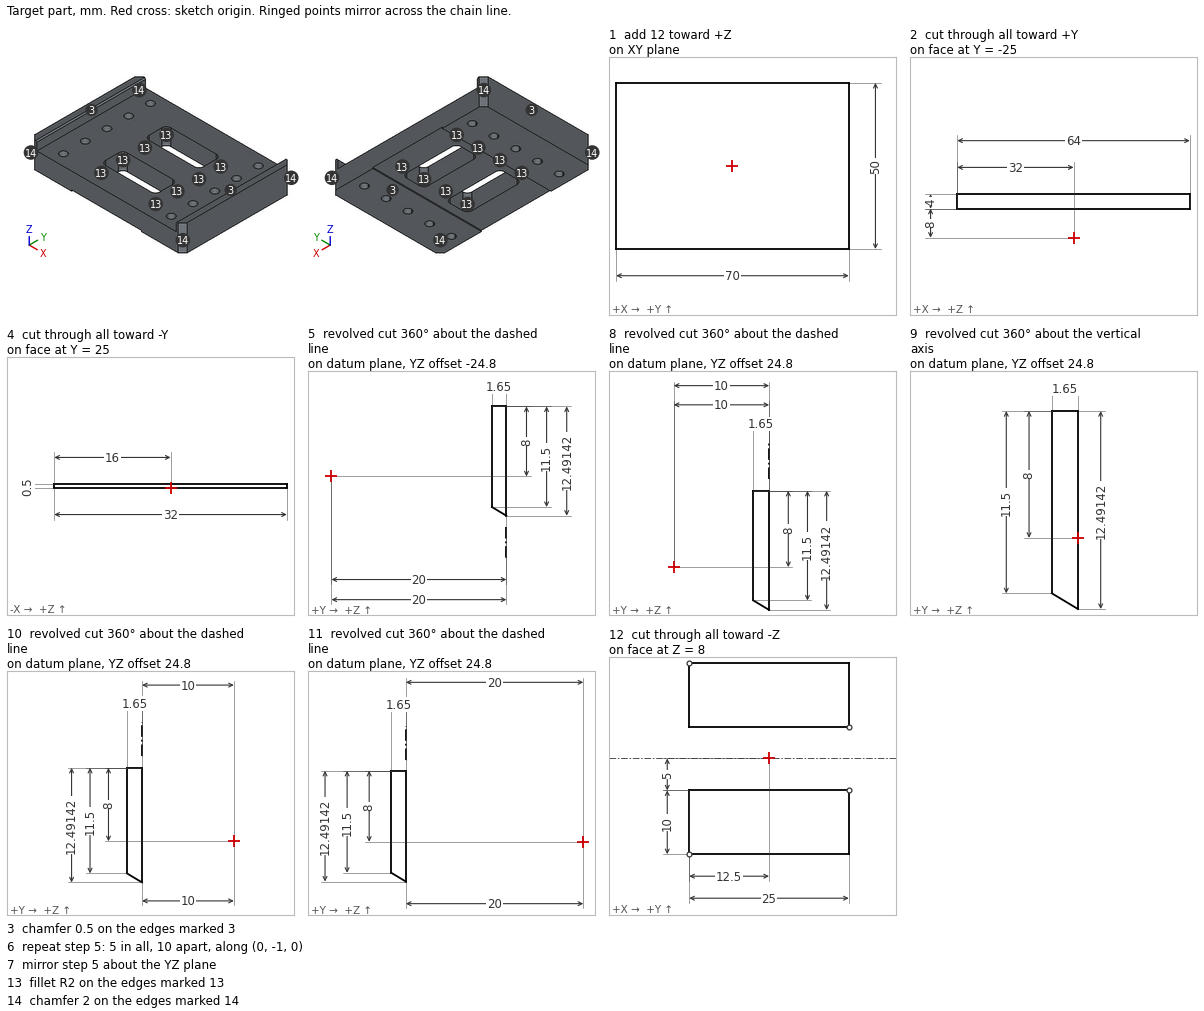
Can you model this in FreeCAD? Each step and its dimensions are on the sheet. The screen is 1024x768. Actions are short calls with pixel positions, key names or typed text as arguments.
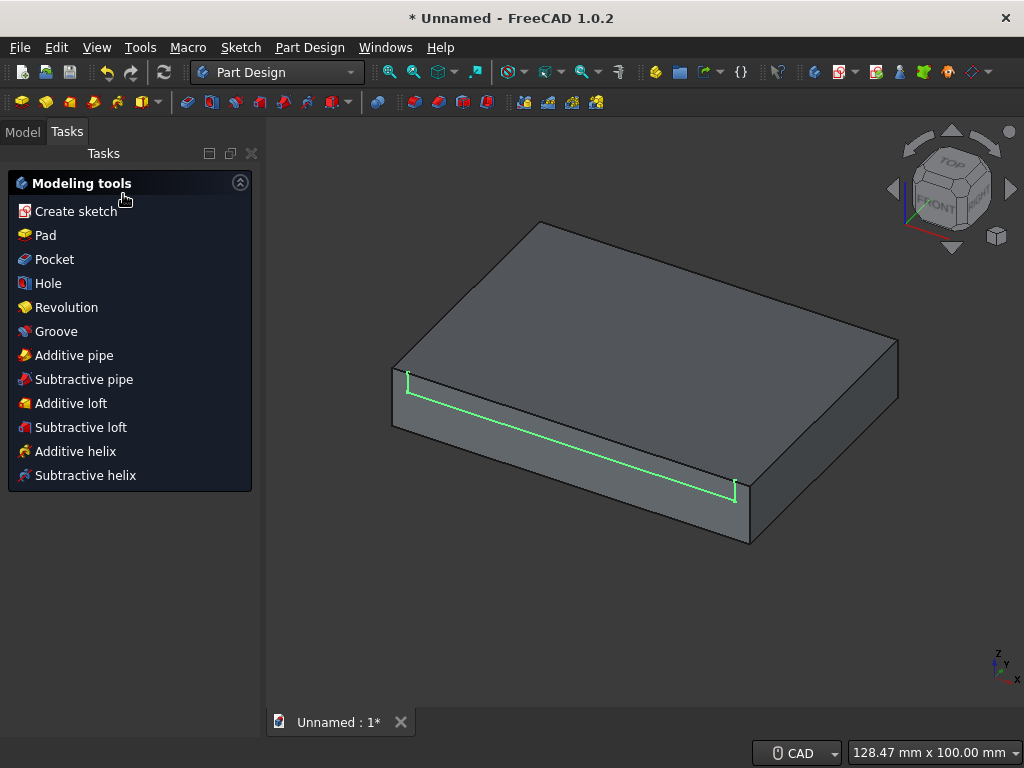
click(188, 102)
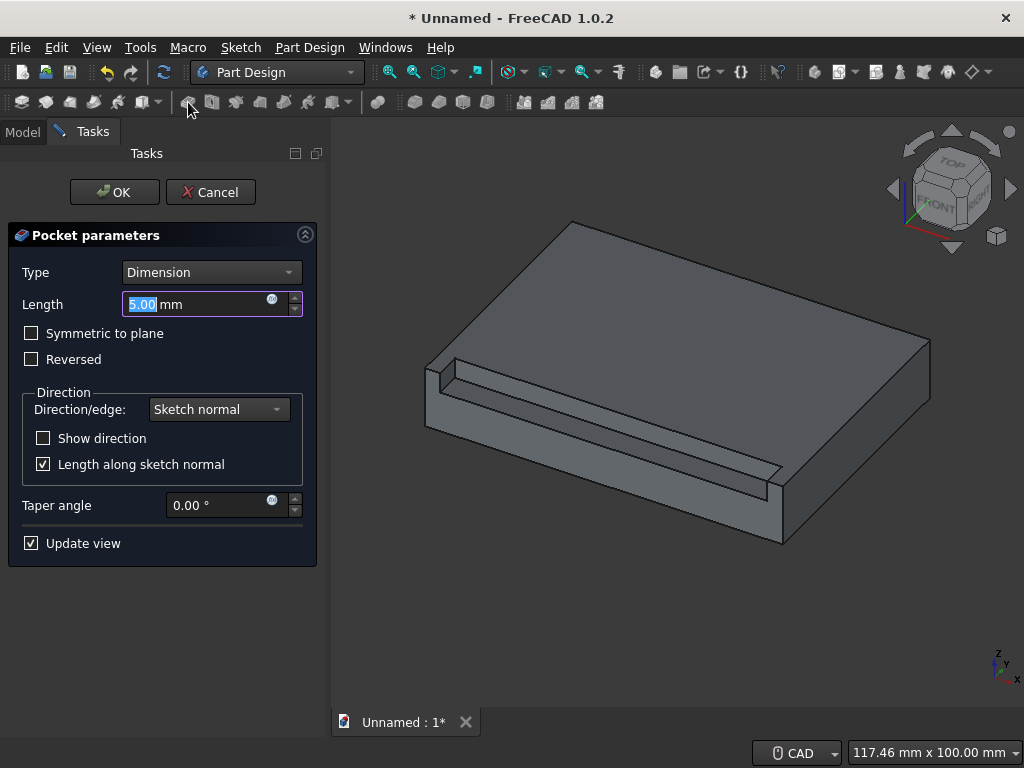
click(212, 272)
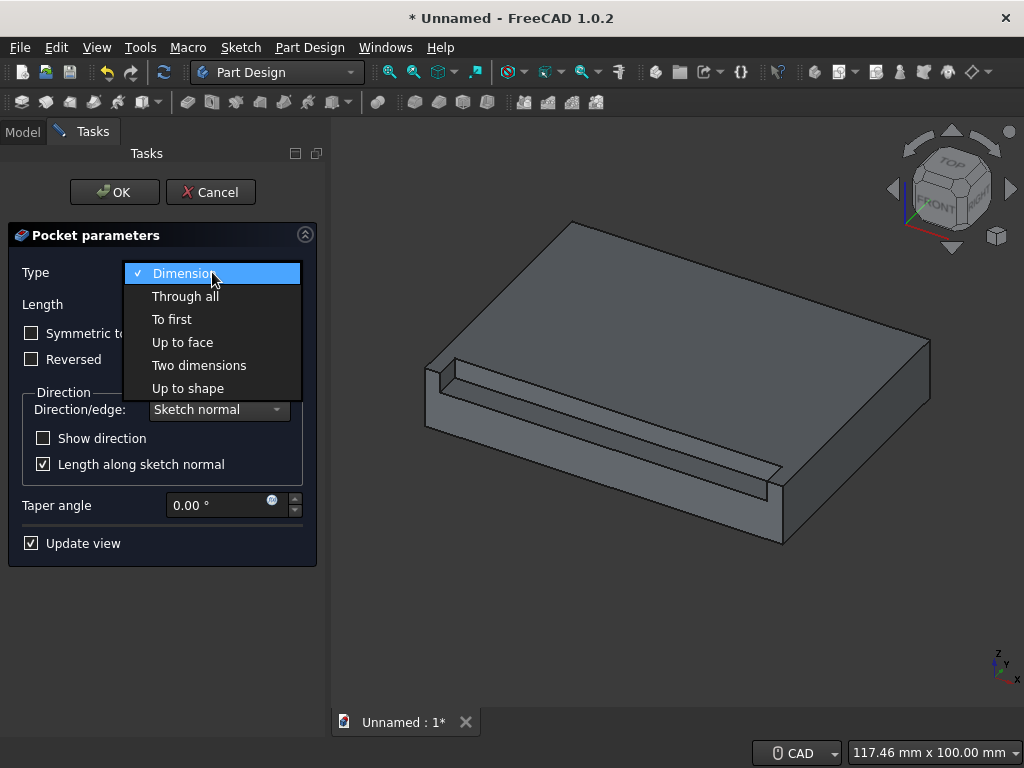
click(212, 296)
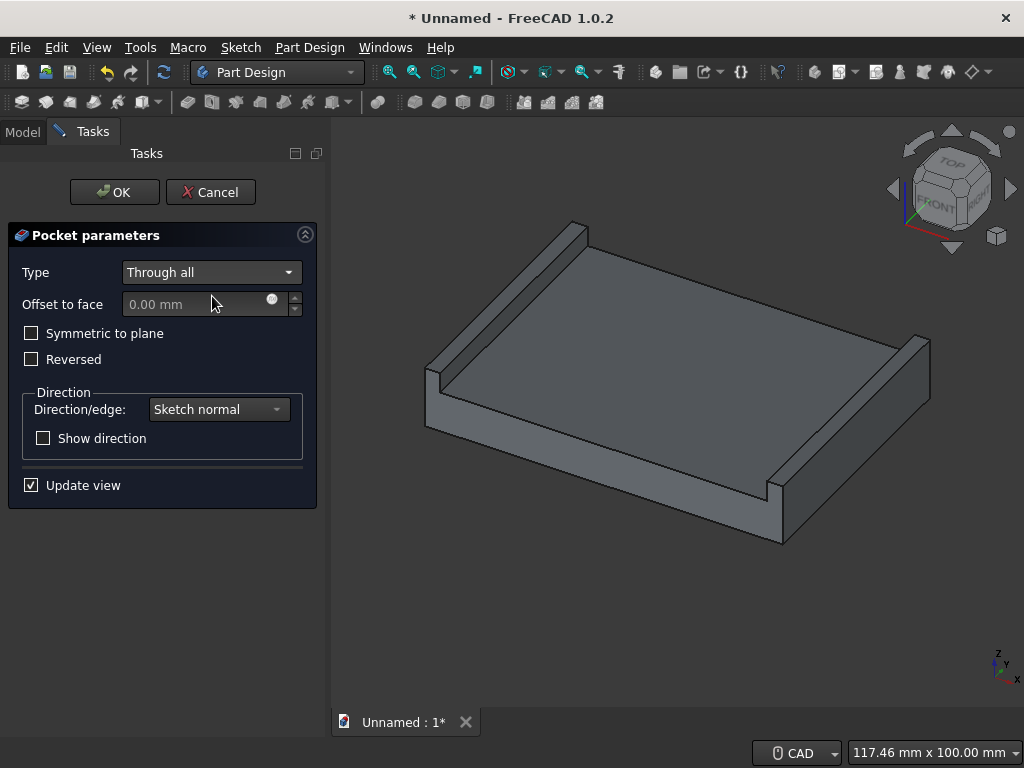
click(115, 192)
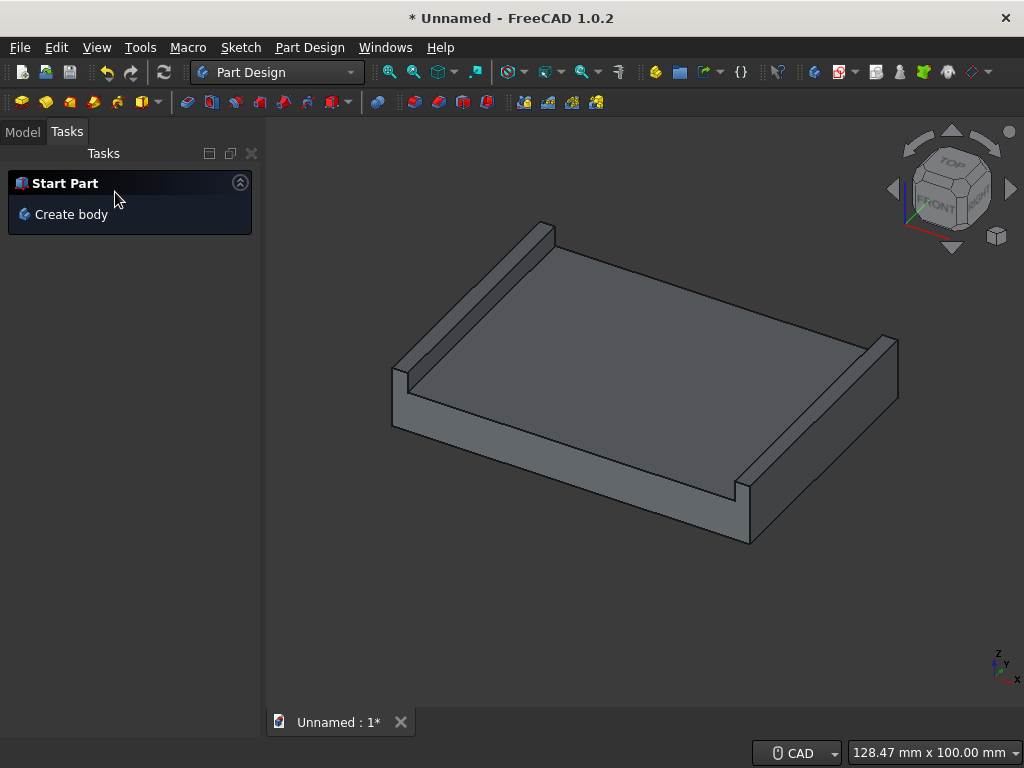
click(481, 299)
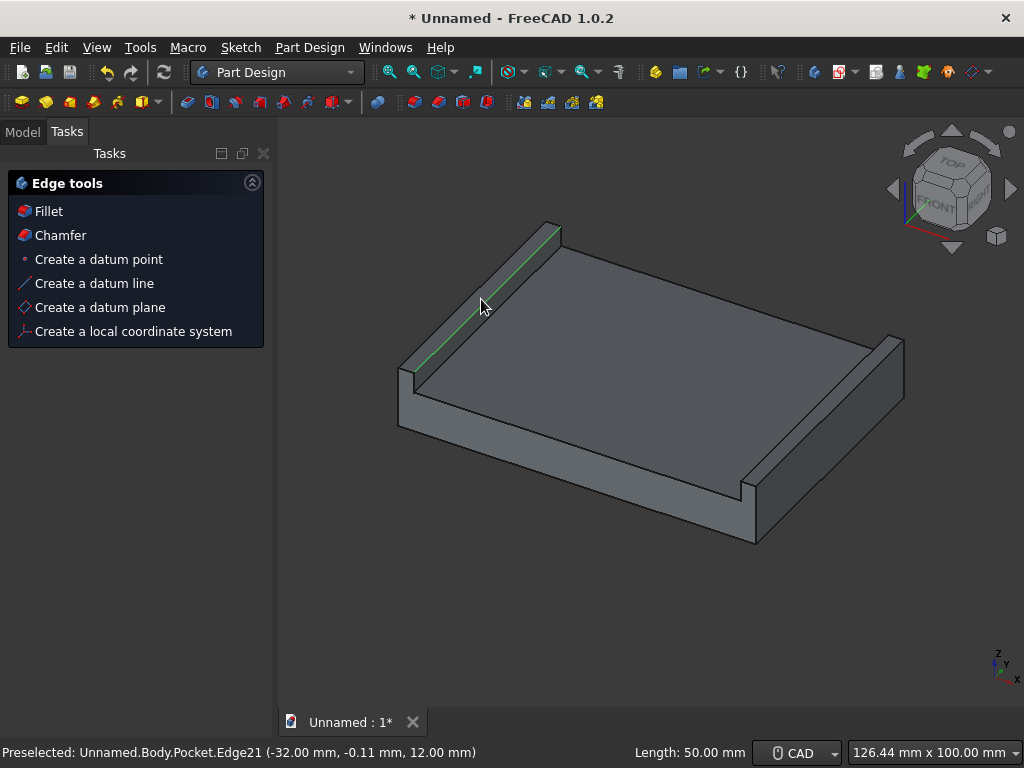
key(0)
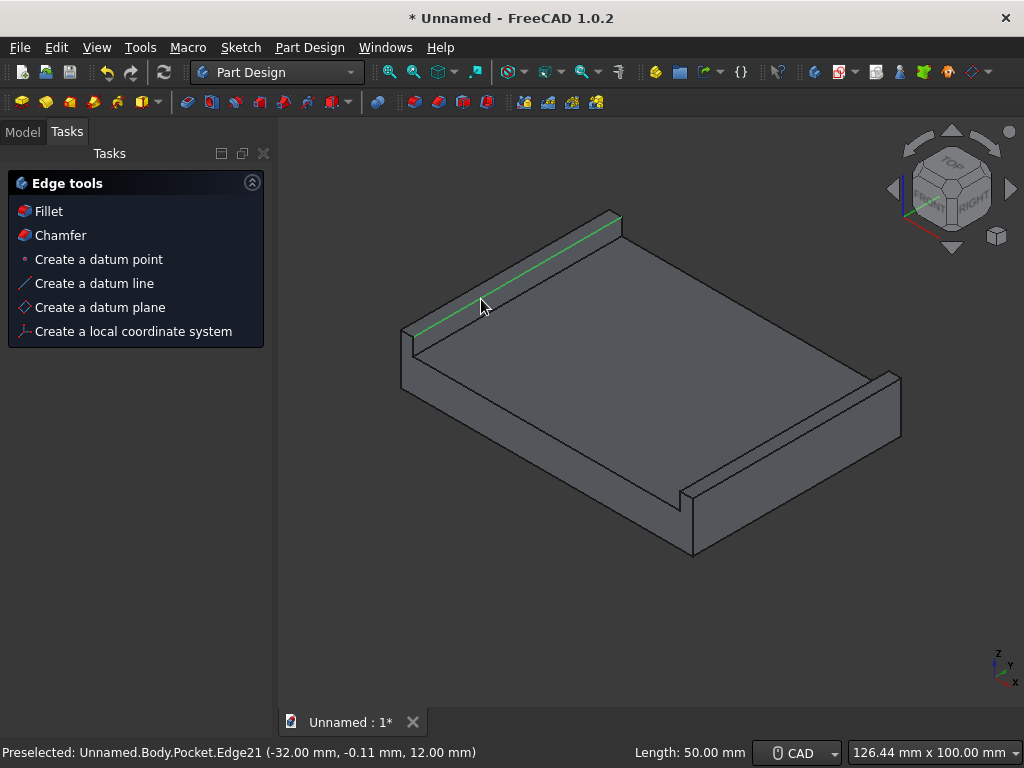
key(2)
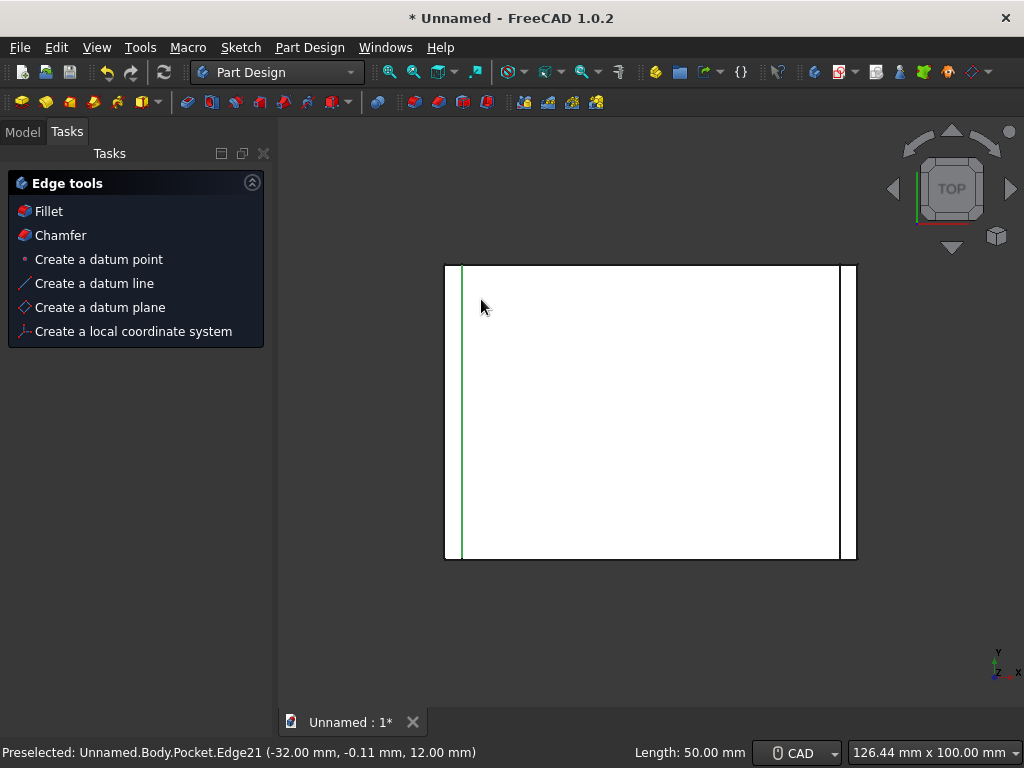
click(840, 411, ctrl)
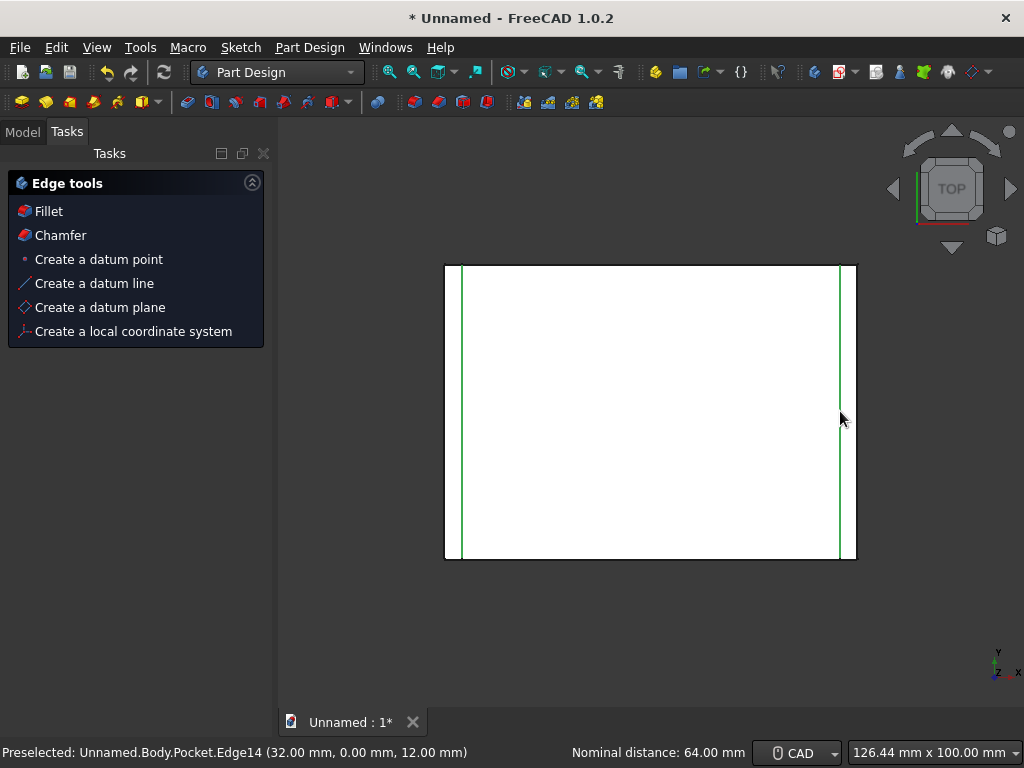
click(440, 102)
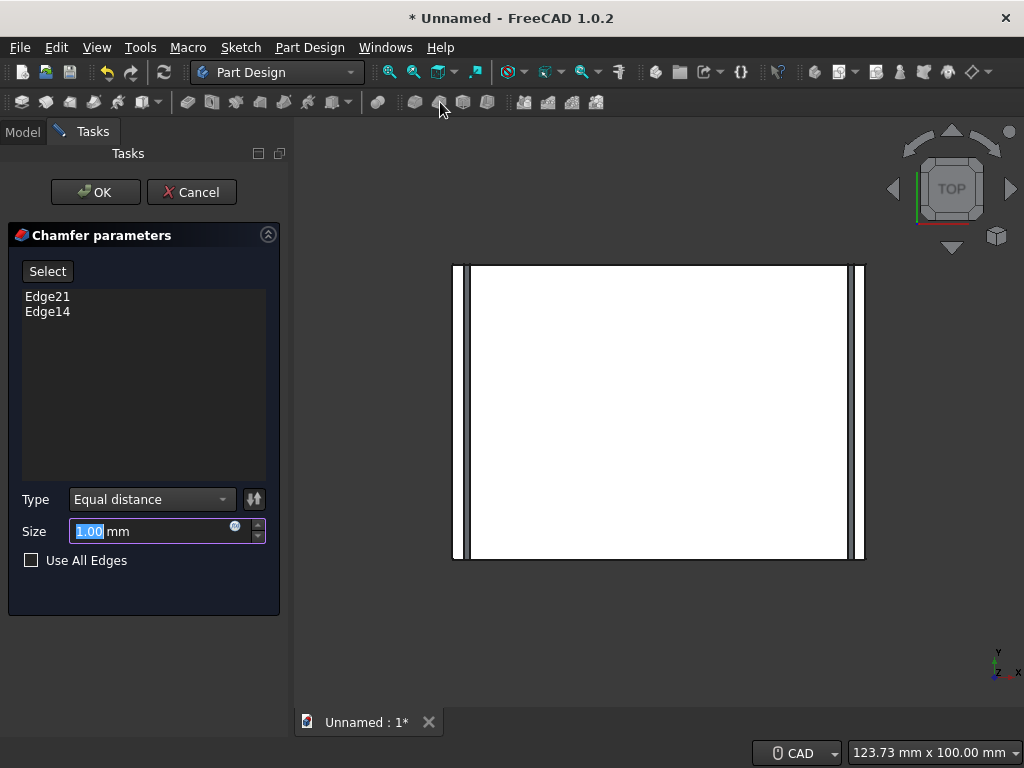
text(0.5)
key(Tab)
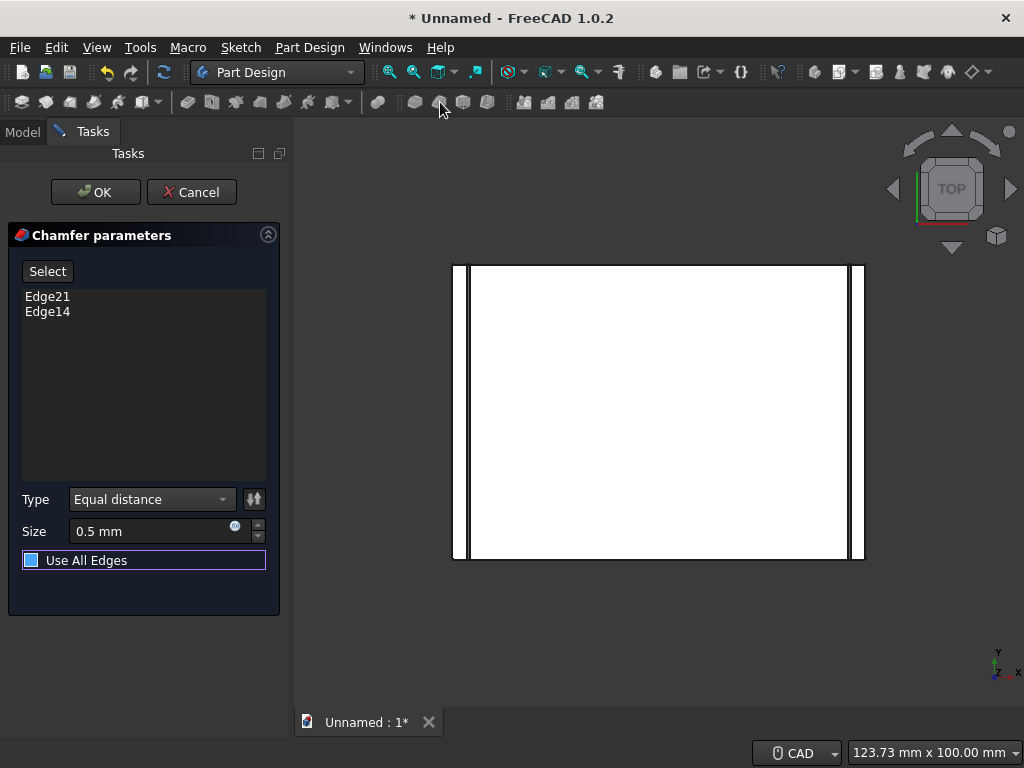
click(96, 192)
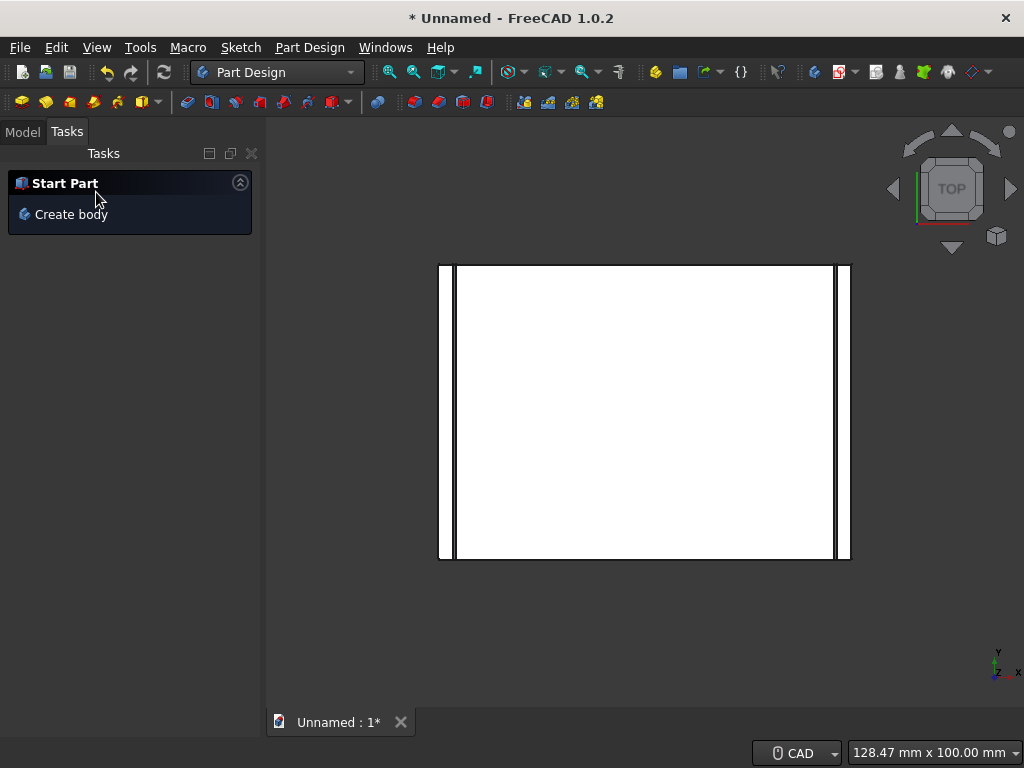
key(4)